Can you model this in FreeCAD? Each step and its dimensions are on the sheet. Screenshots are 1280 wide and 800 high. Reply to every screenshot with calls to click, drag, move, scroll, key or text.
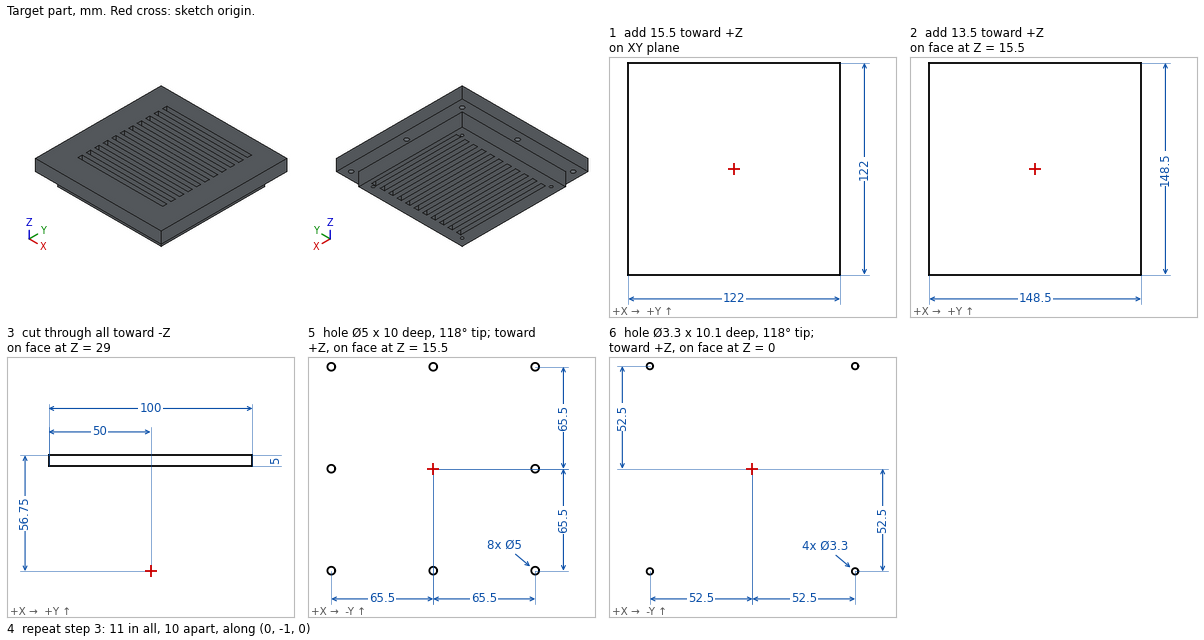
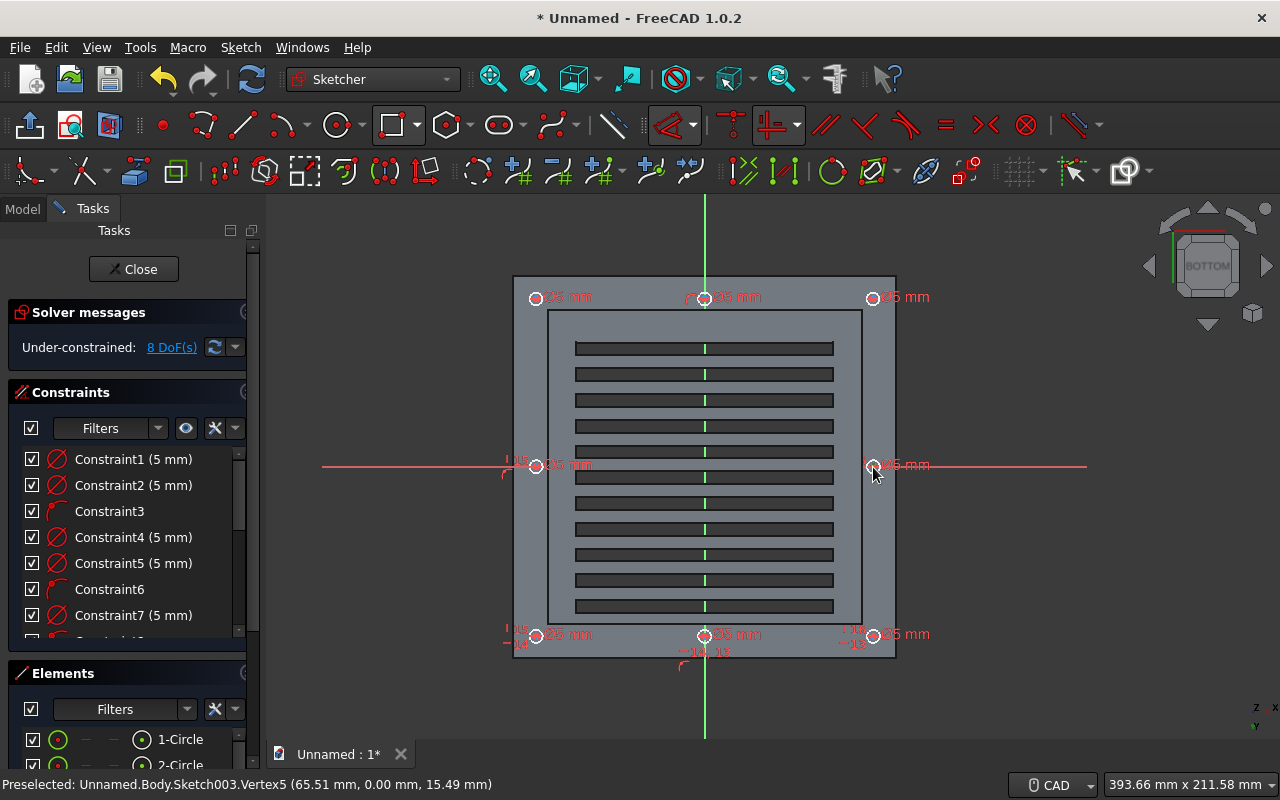
click(873, 299)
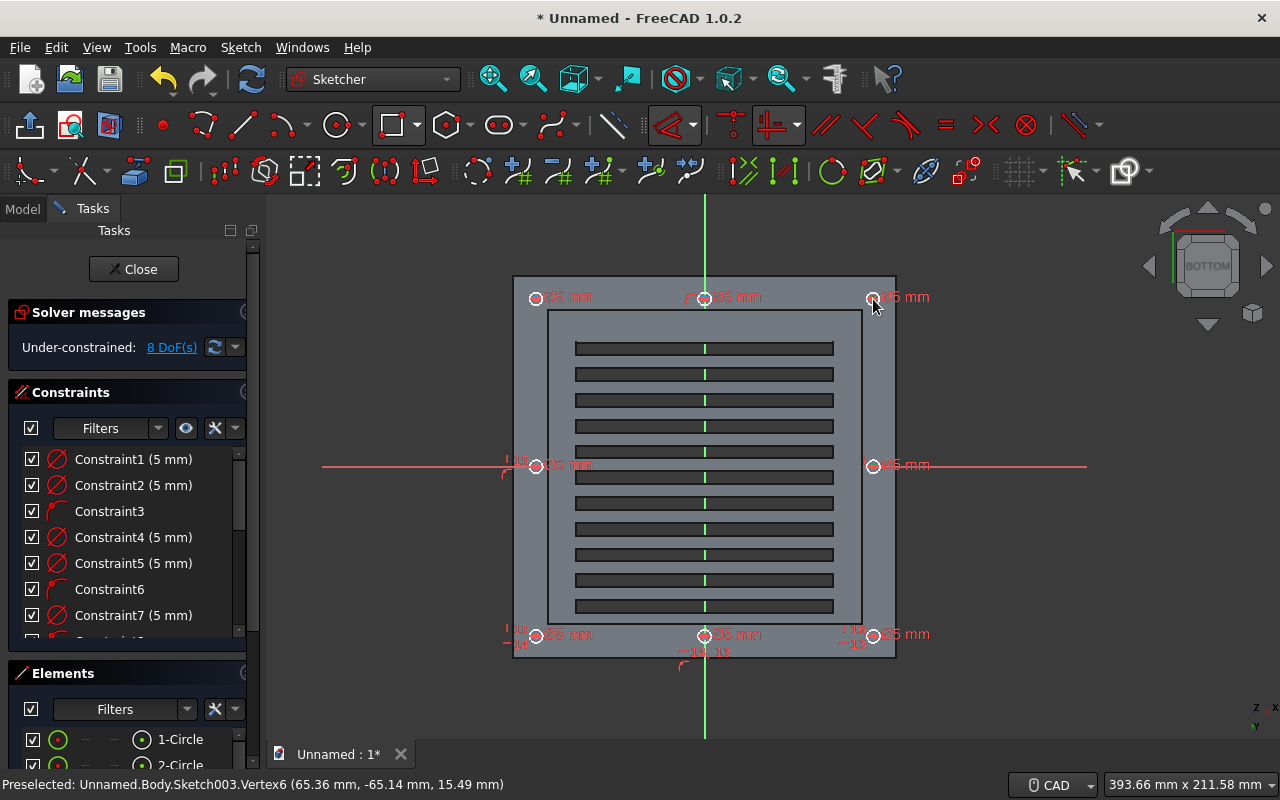
key(v)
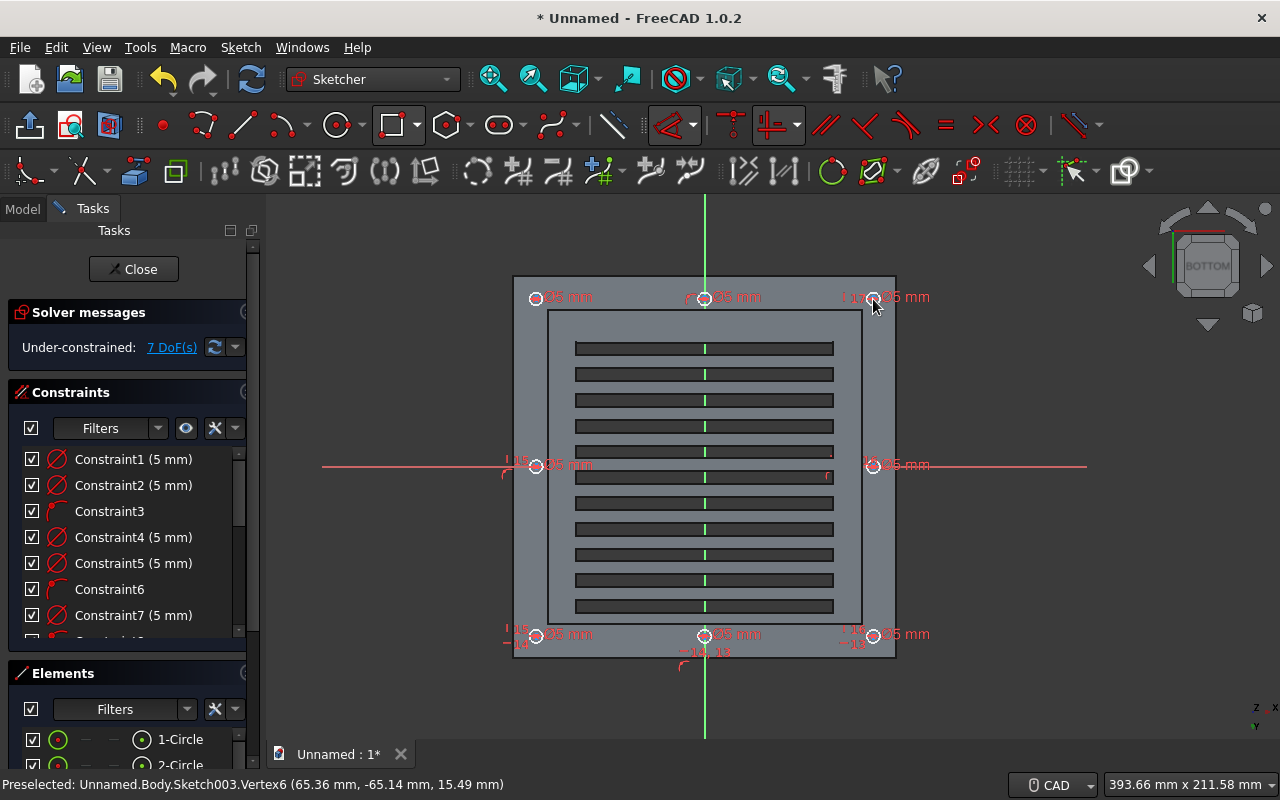
click(873, 299)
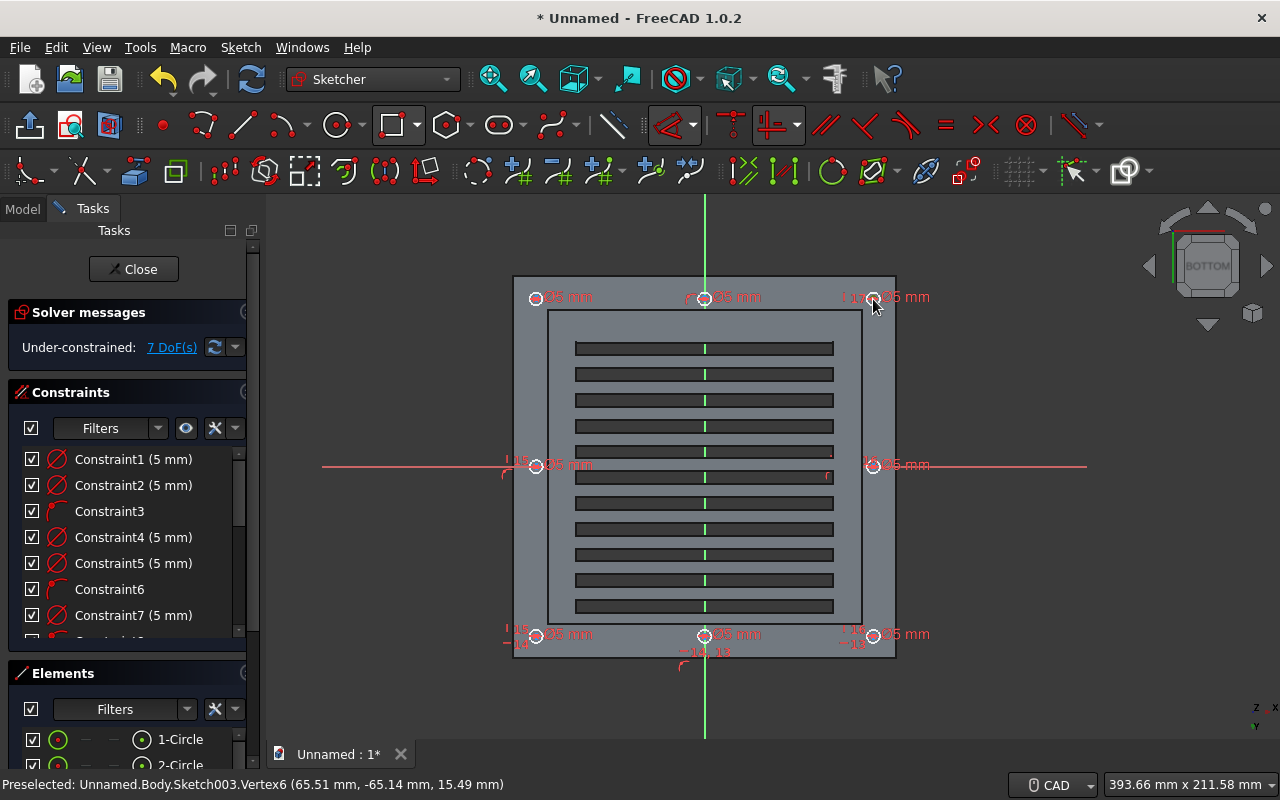
click(705, 299)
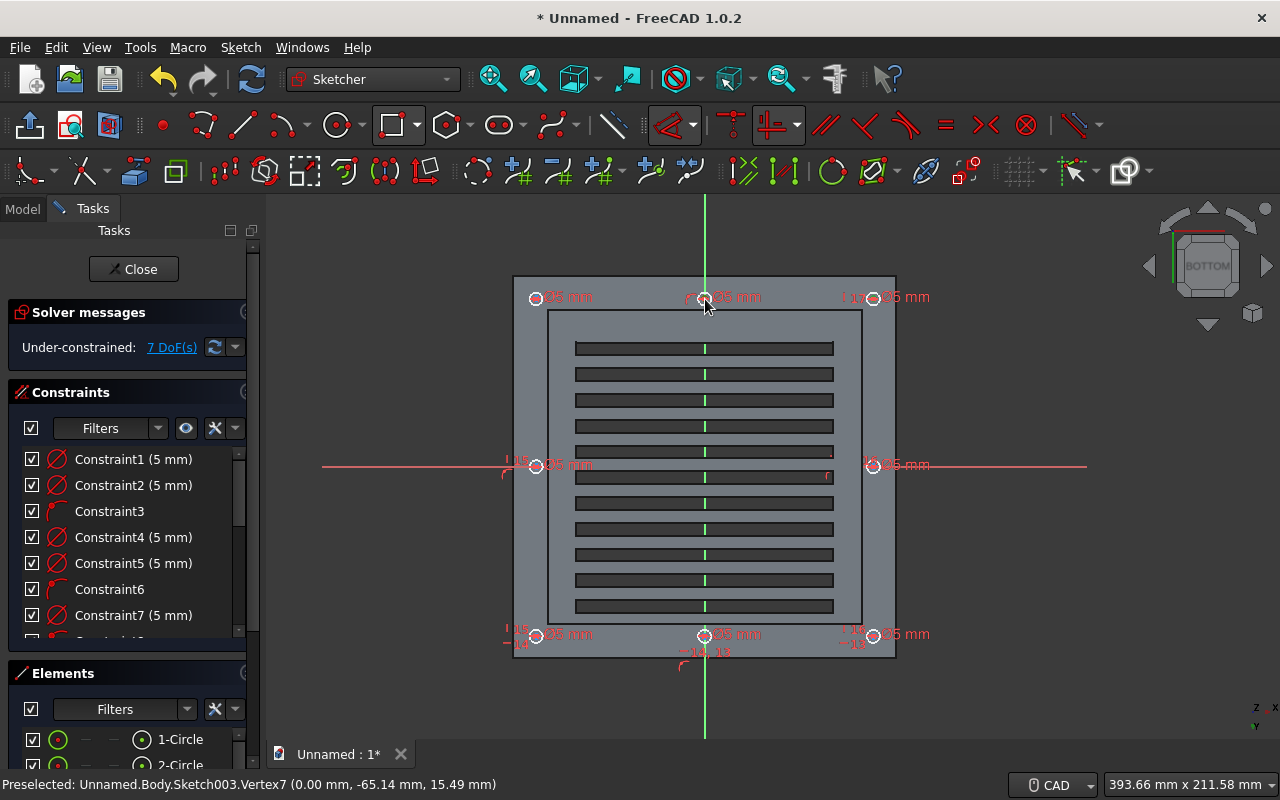
click(800, 126)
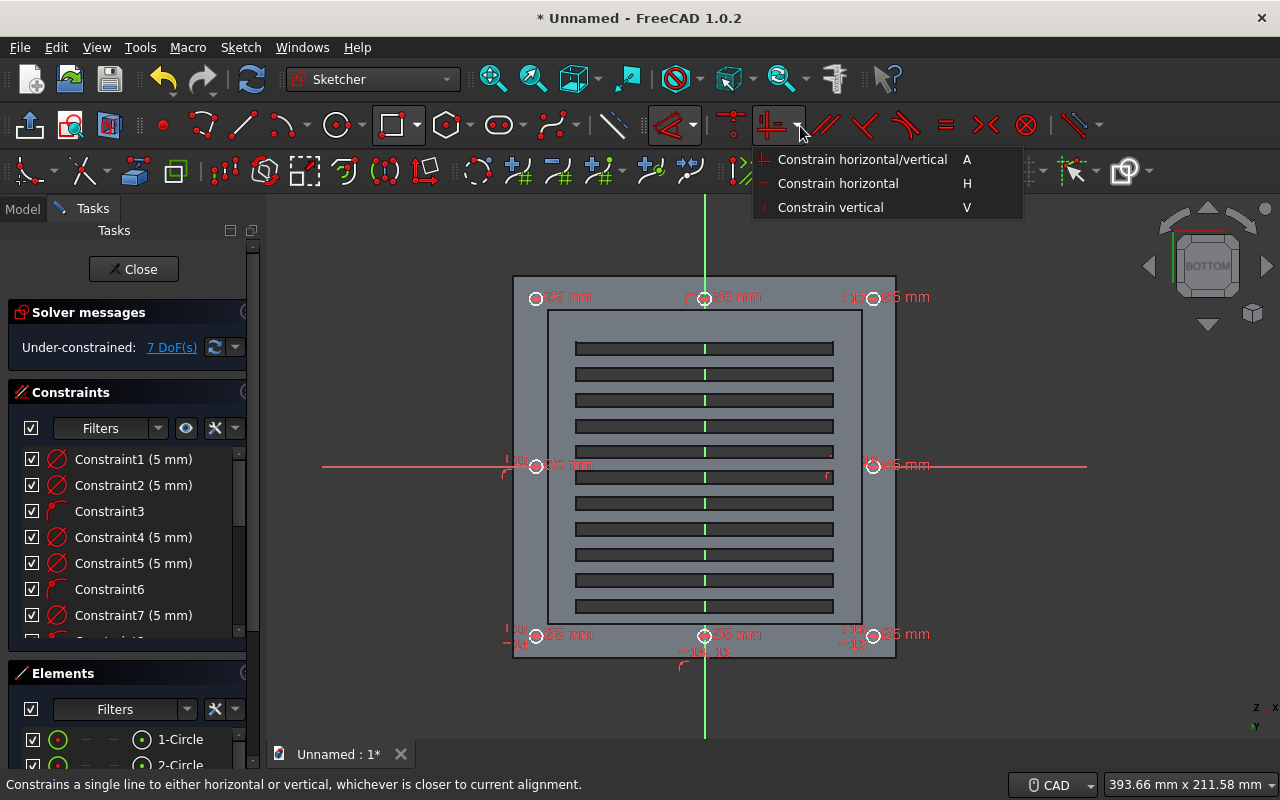
click(888, 183)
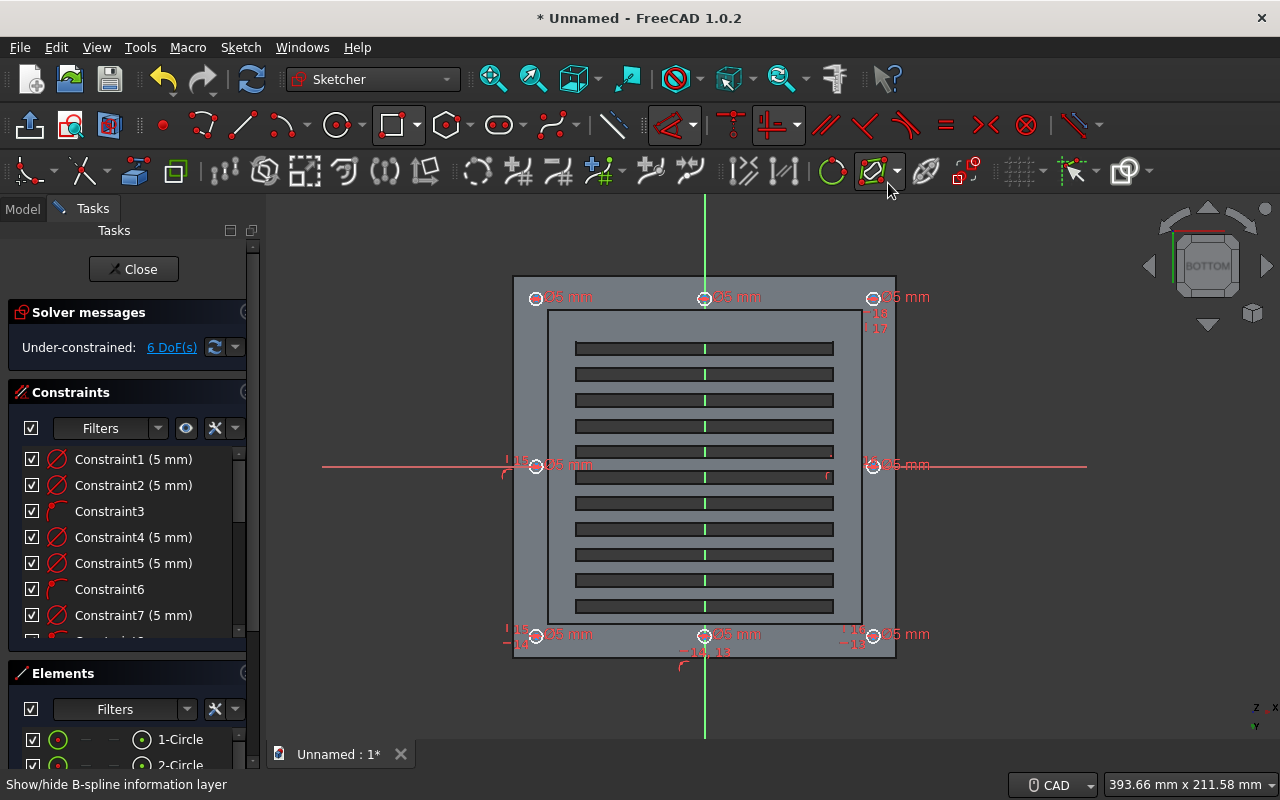
click(536, 467)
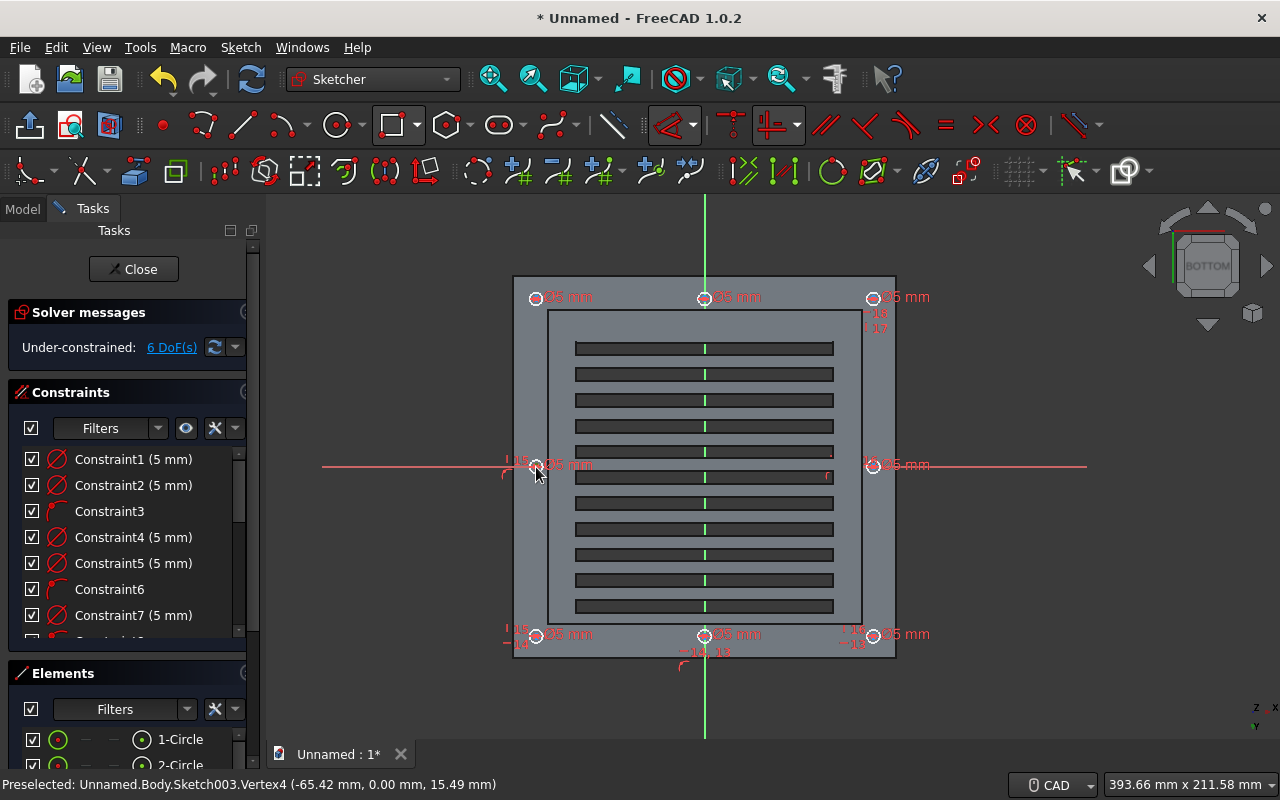
click(536, 299)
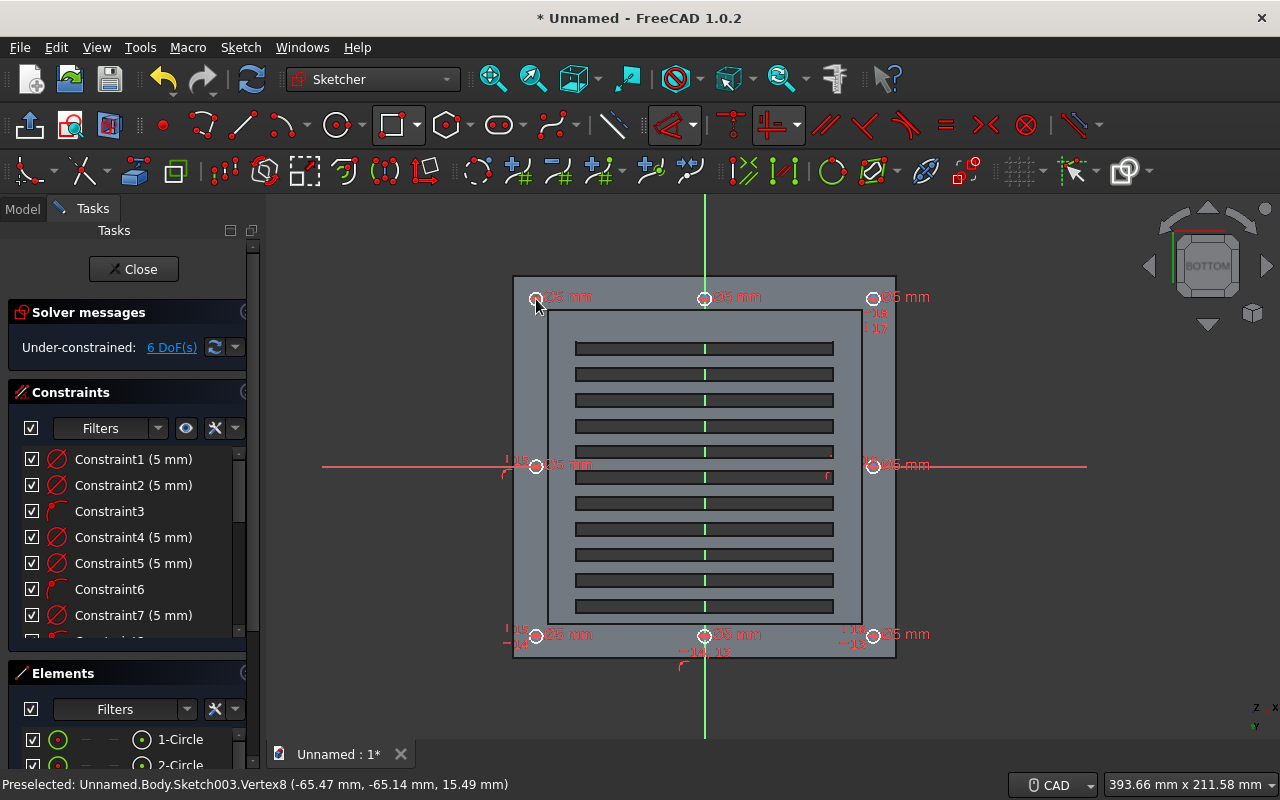
click(800, 126)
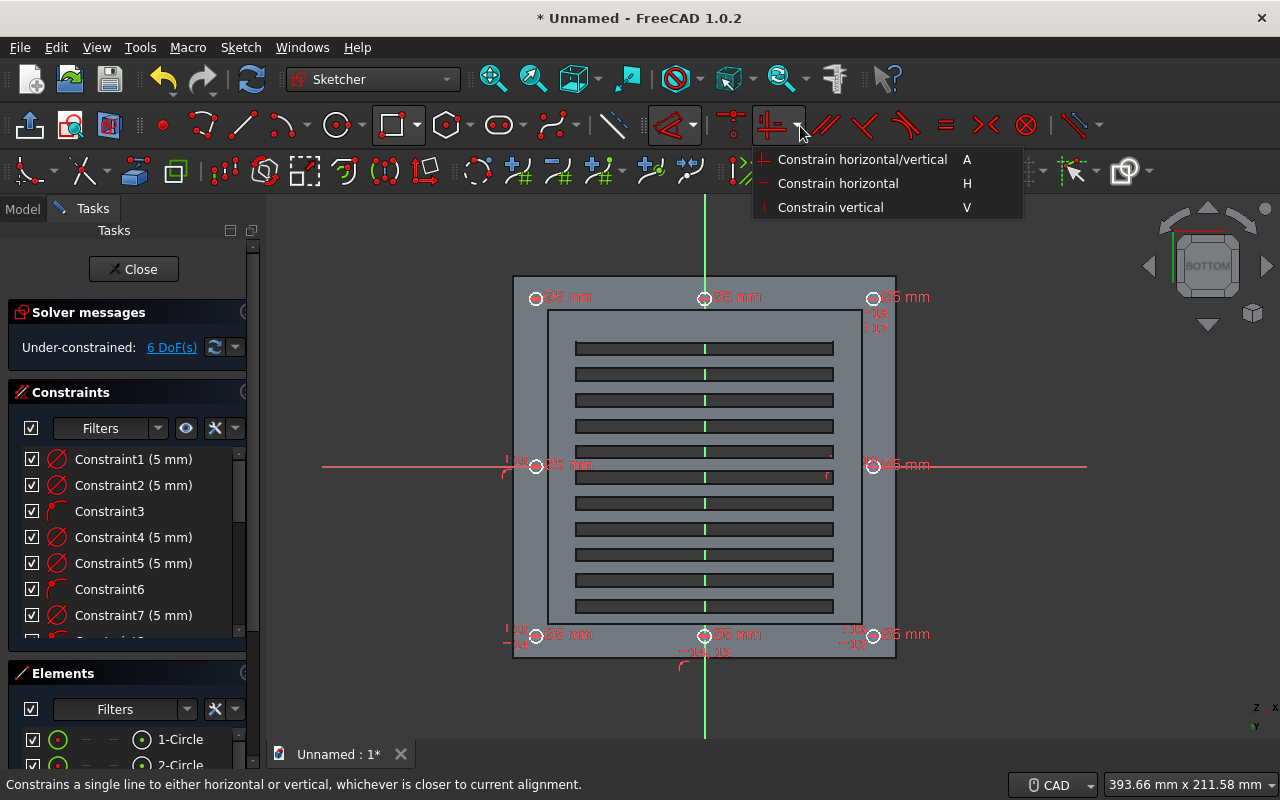
click(888, 207)